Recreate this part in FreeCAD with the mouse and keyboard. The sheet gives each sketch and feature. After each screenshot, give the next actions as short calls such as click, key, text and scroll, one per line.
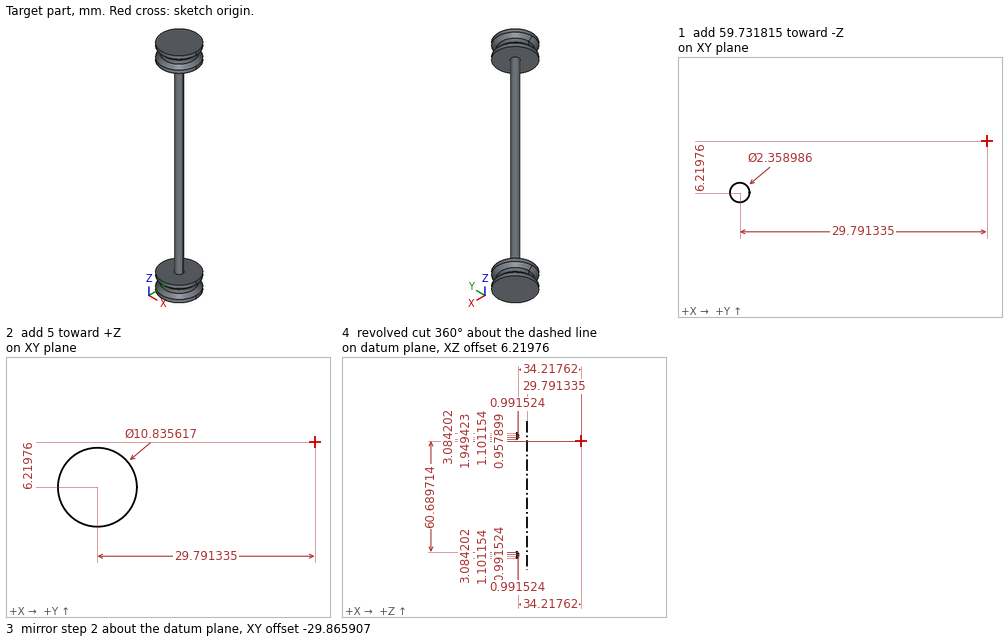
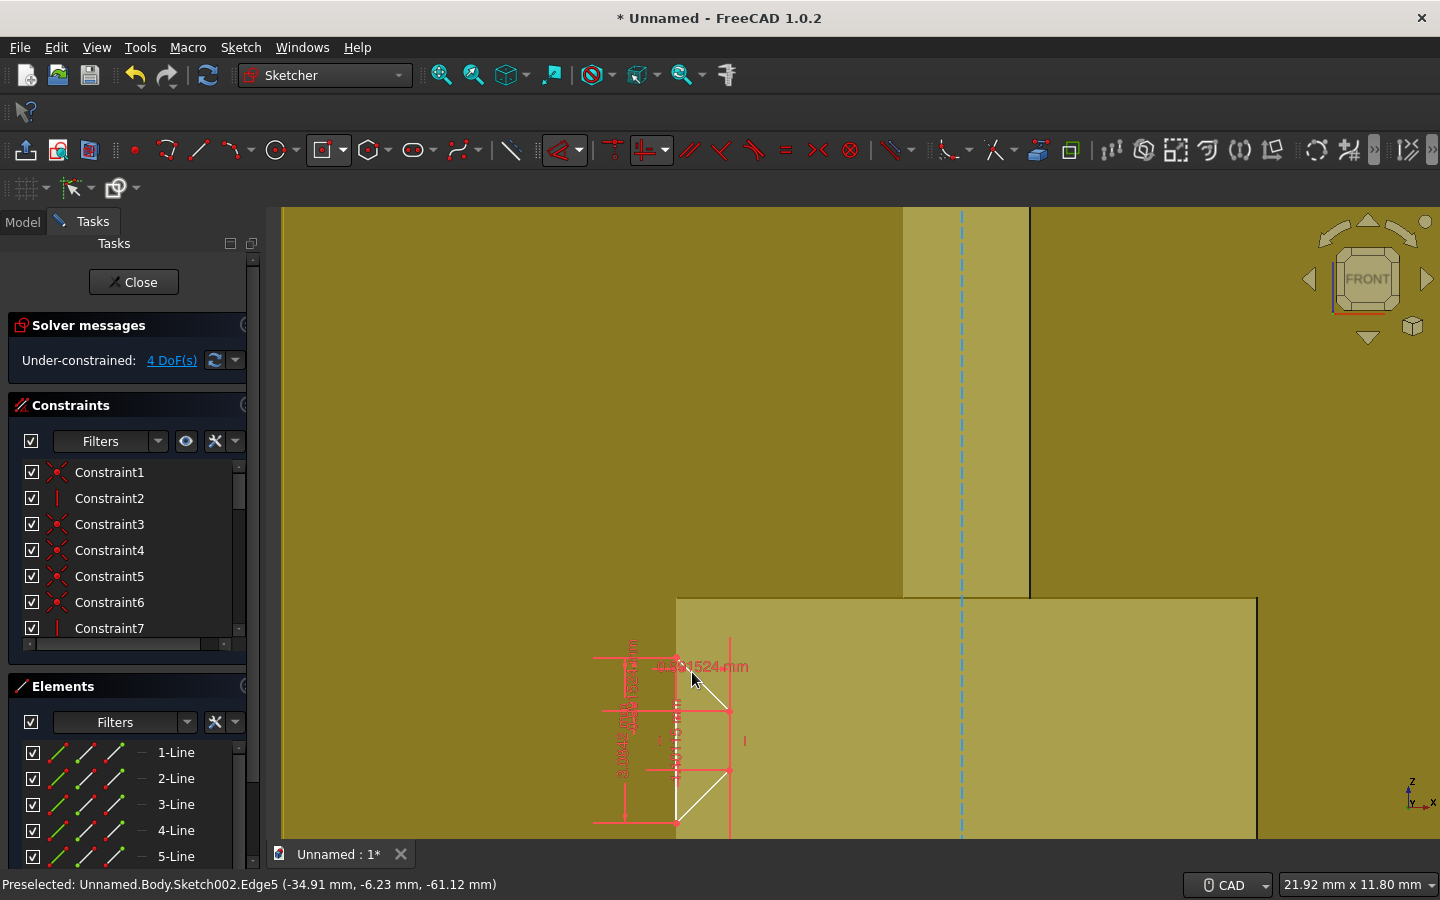
scroll(701, 675, down, 12)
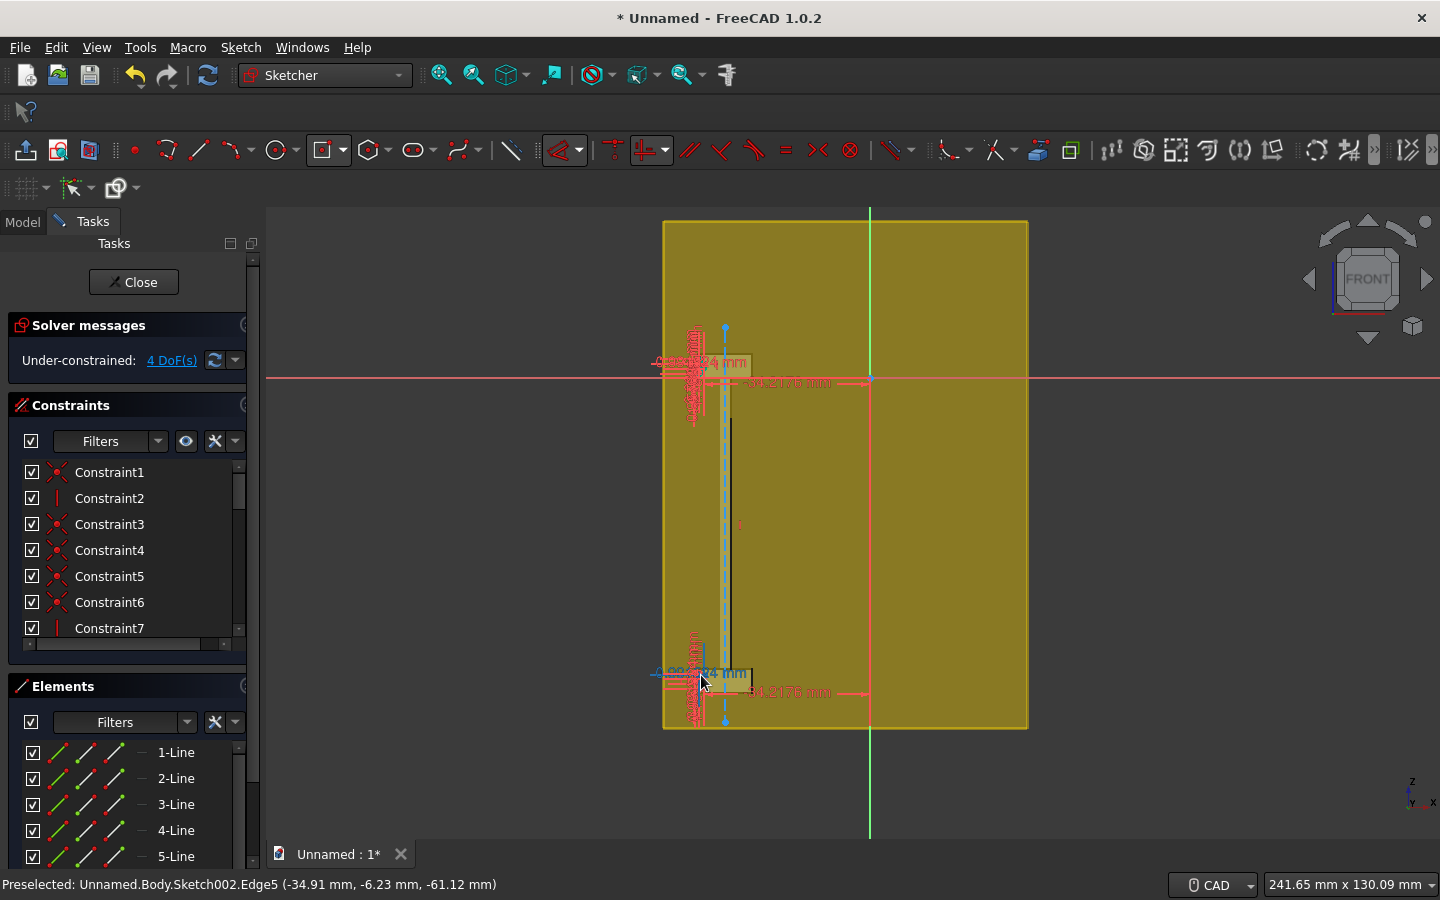
scroll(699, 674, up, 3)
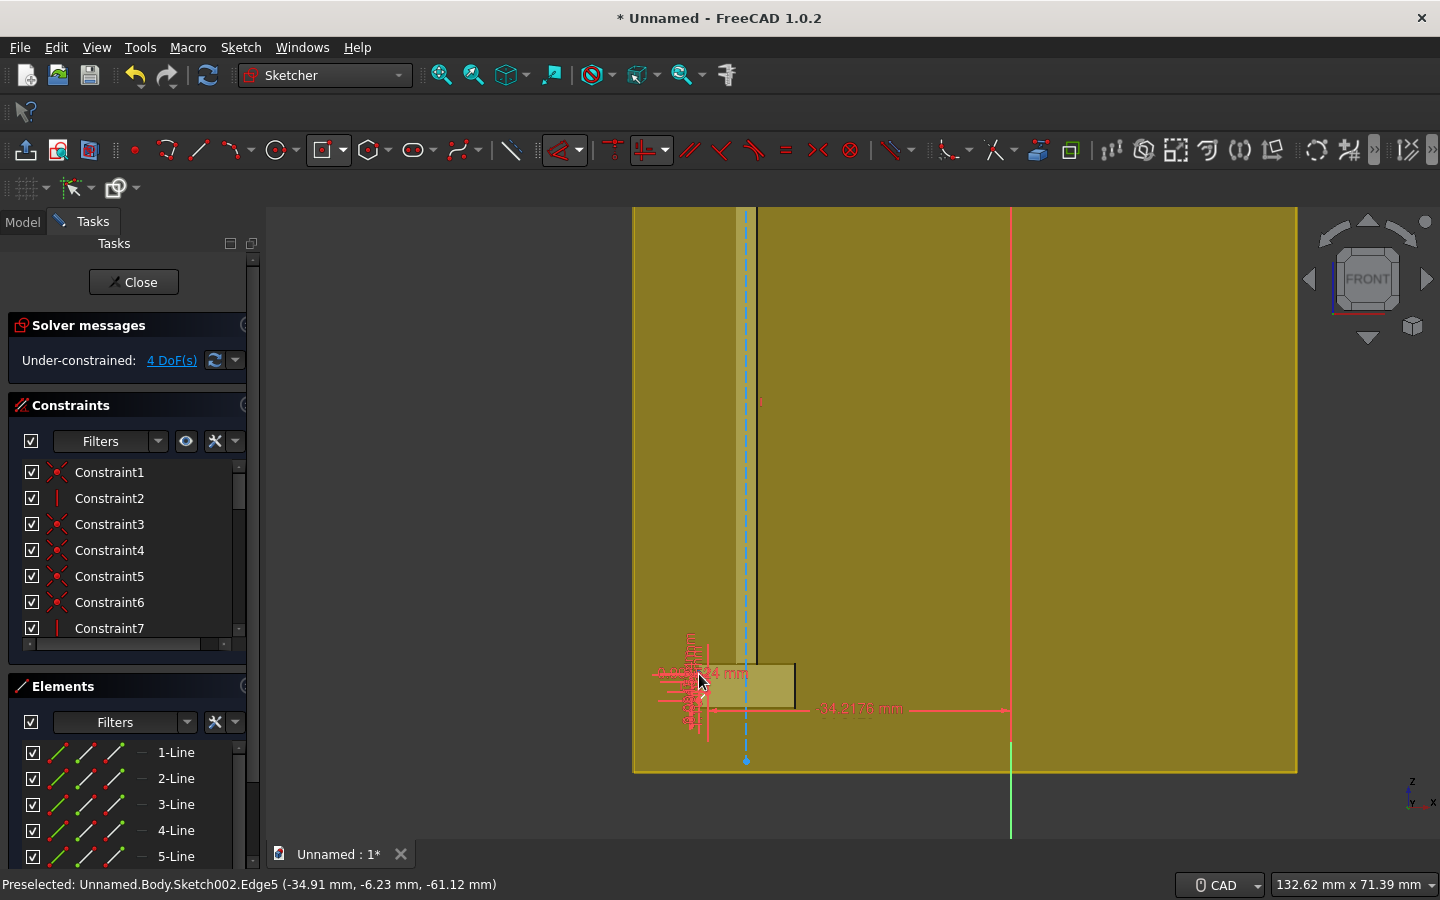
click(699, 674)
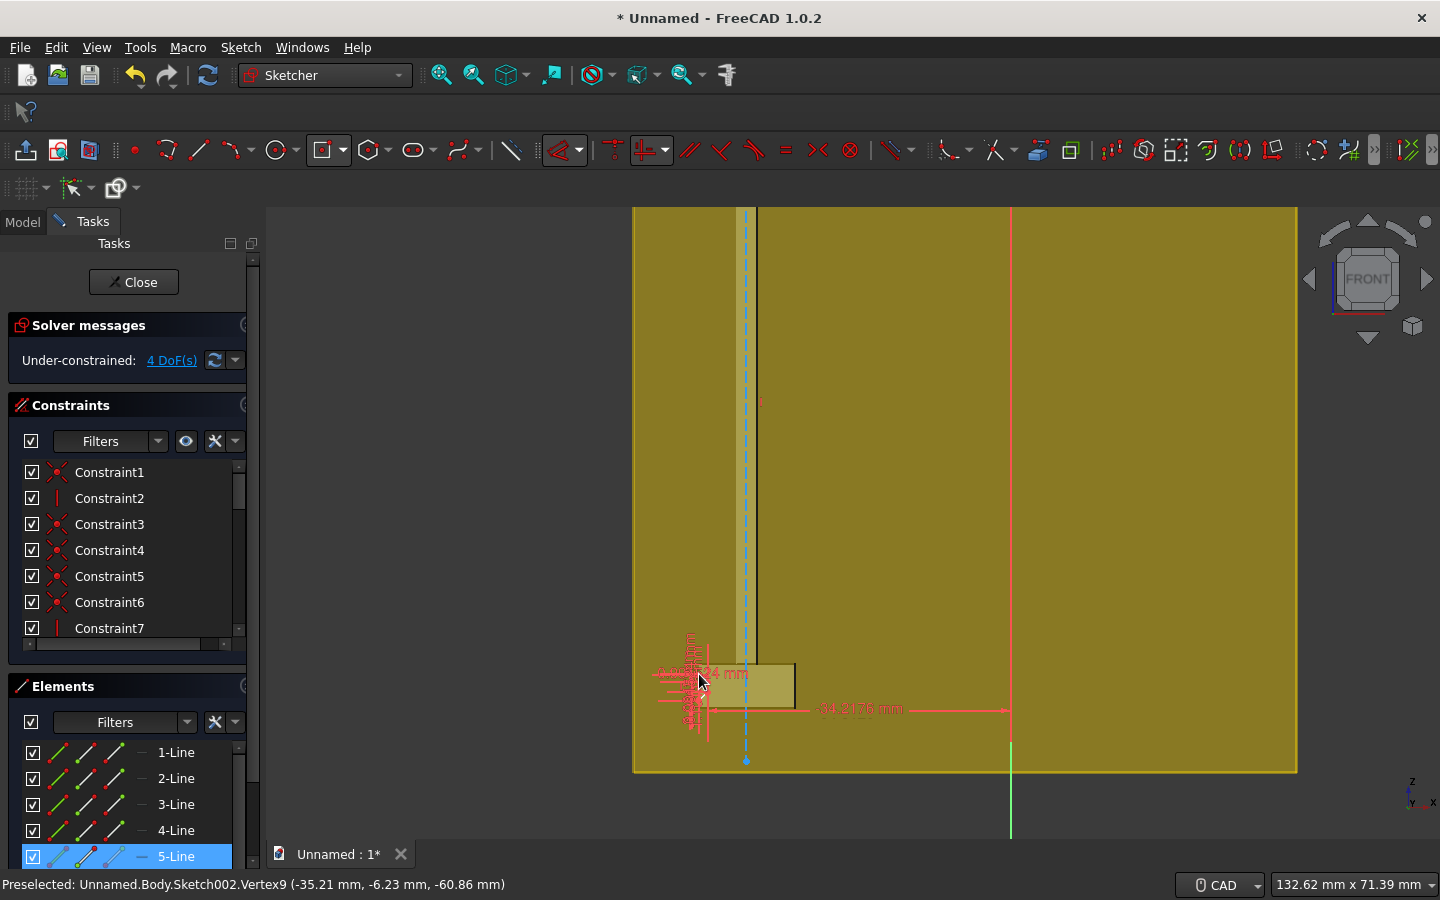
key(i)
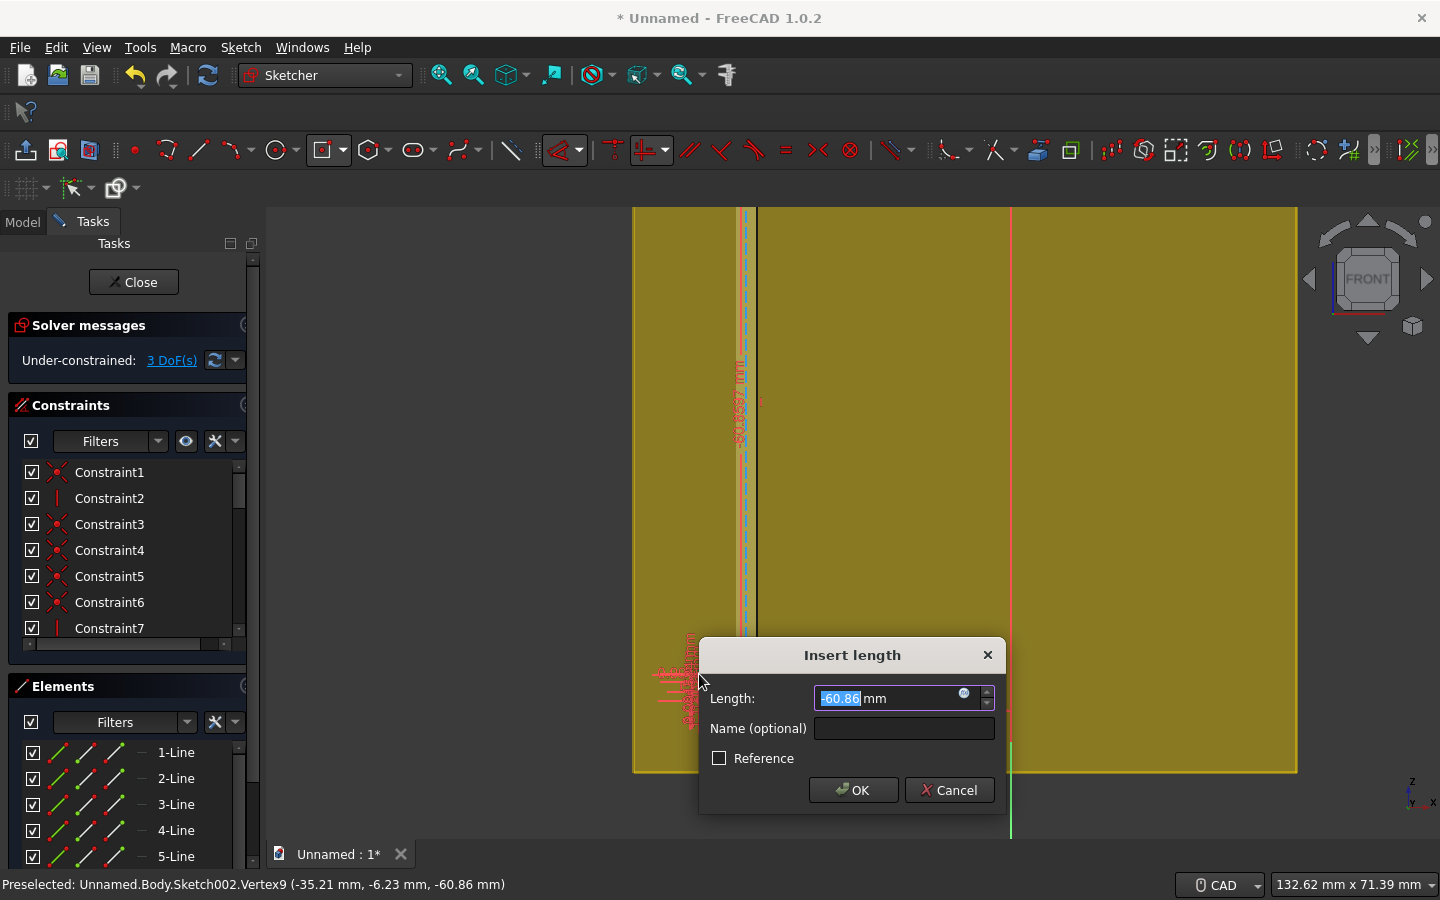
text(-60.689714)
key(Return)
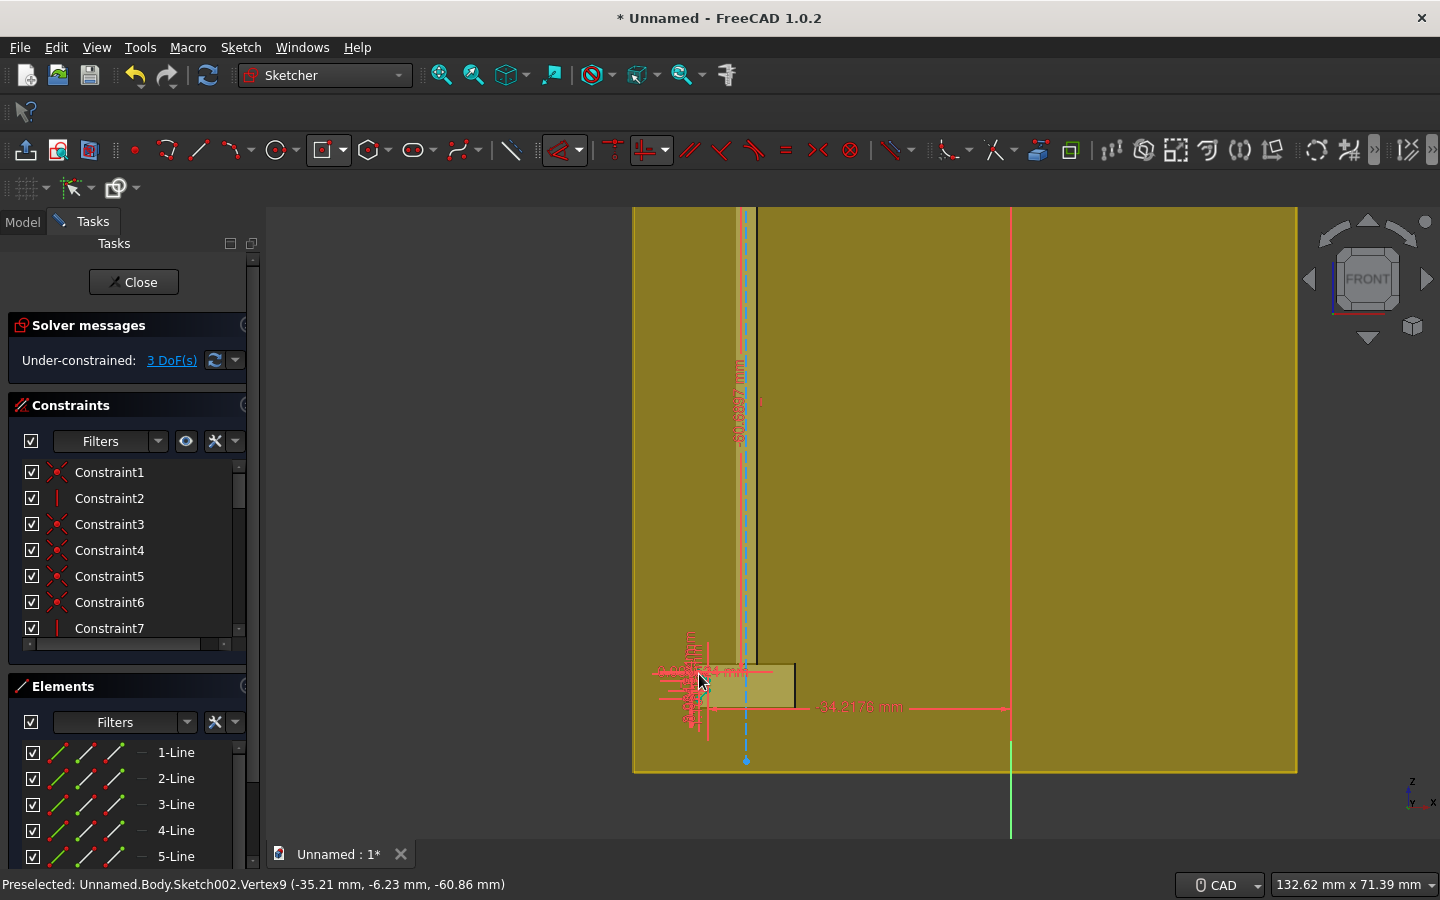
scroll(699, 674, down, 3)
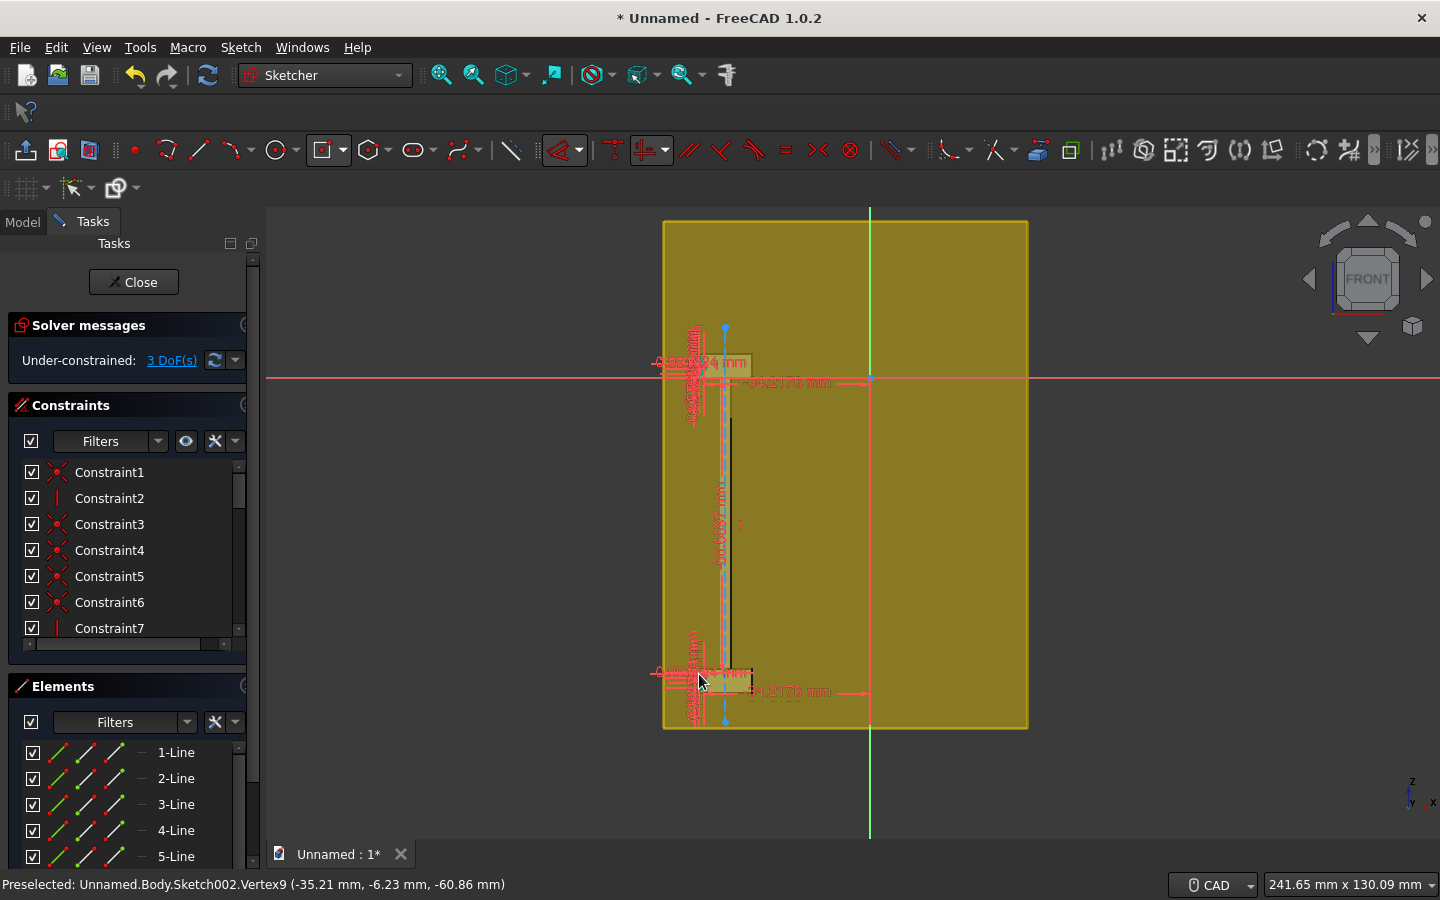
click(725, 327)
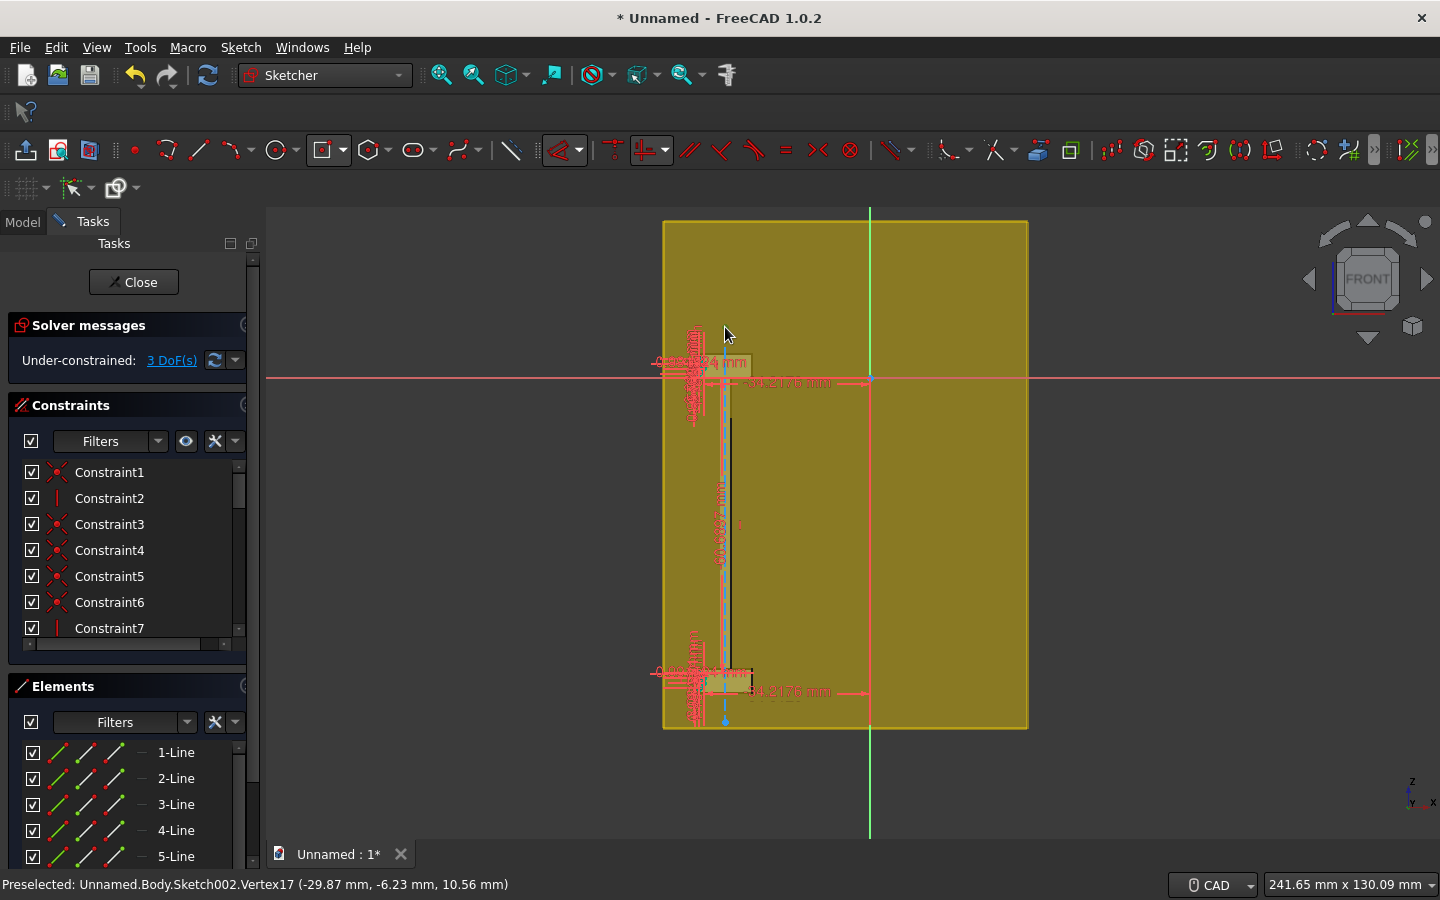
key(l)